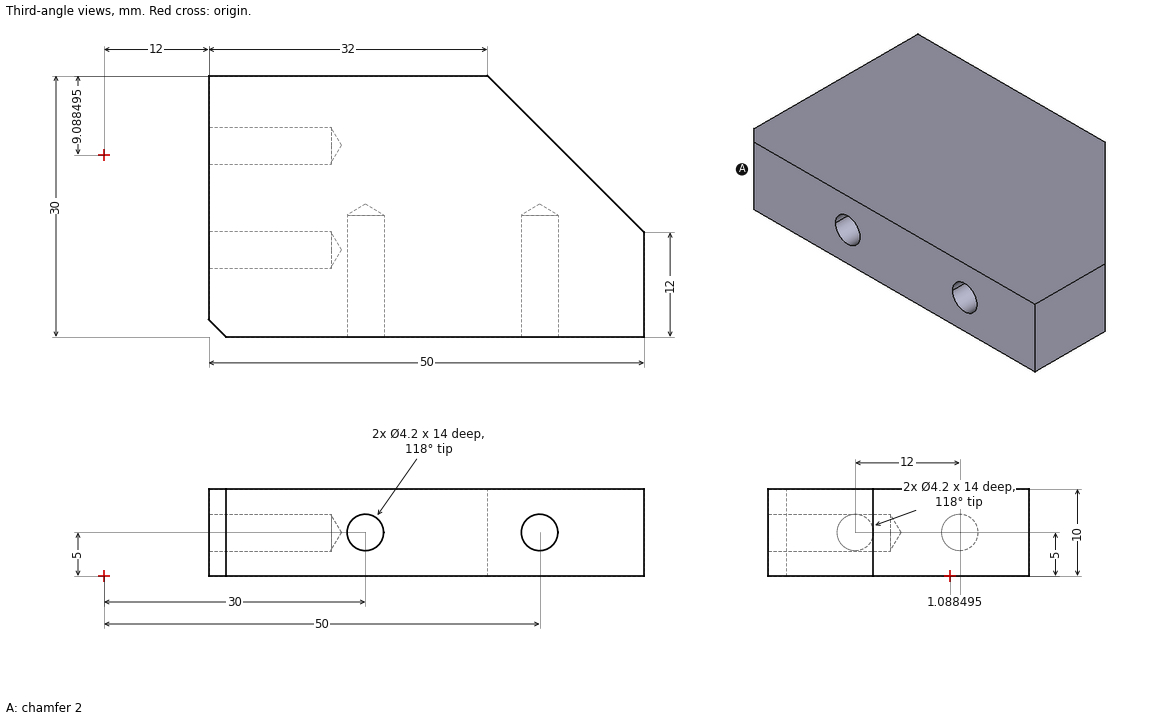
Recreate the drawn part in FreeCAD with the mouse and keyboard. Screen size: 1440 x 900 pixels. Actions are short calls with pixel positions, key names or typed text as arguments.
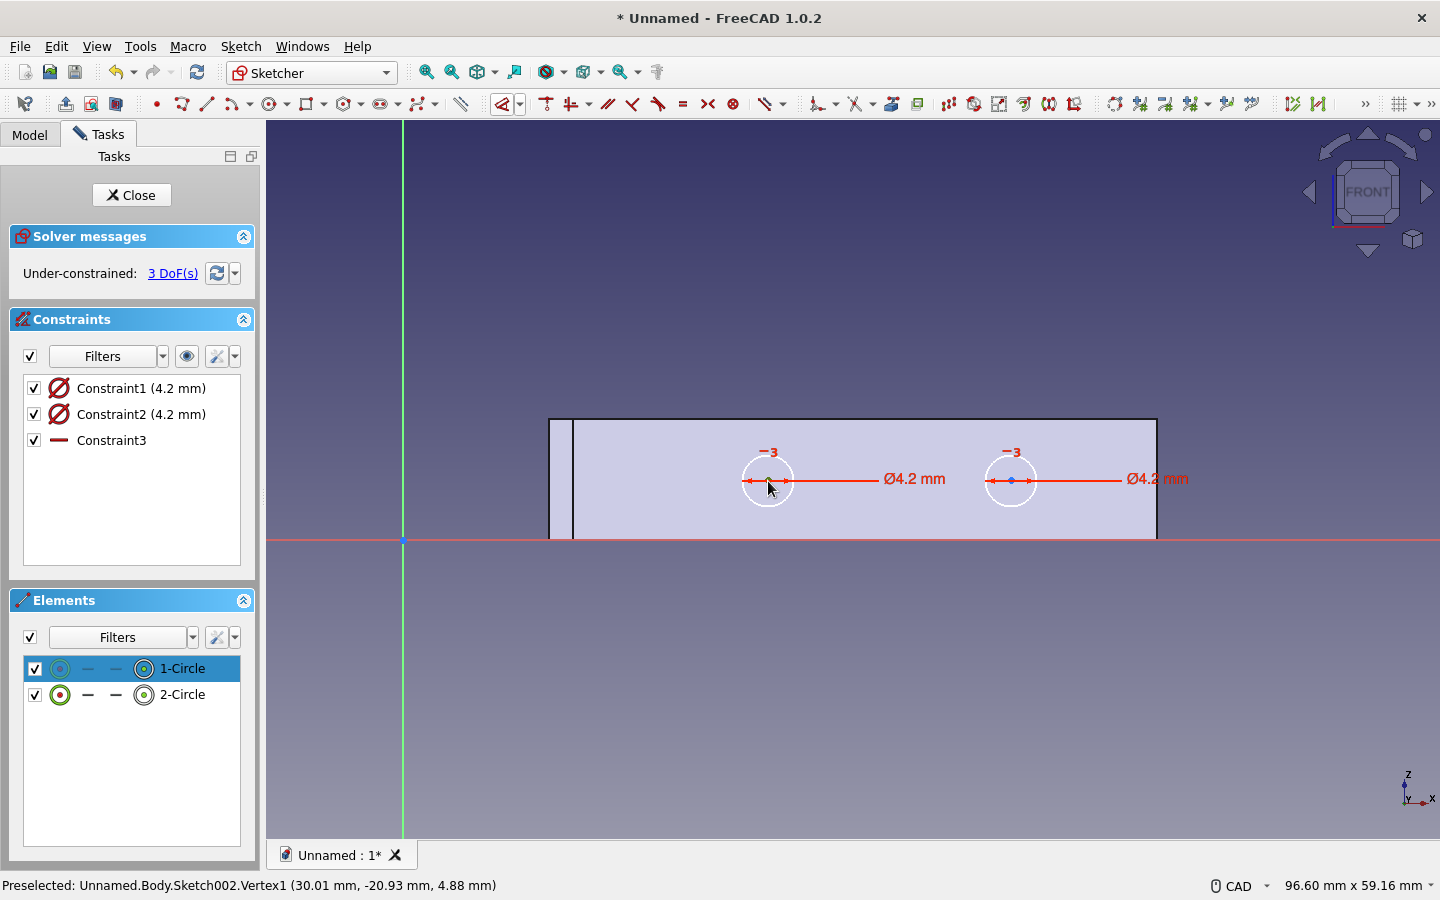
key(i)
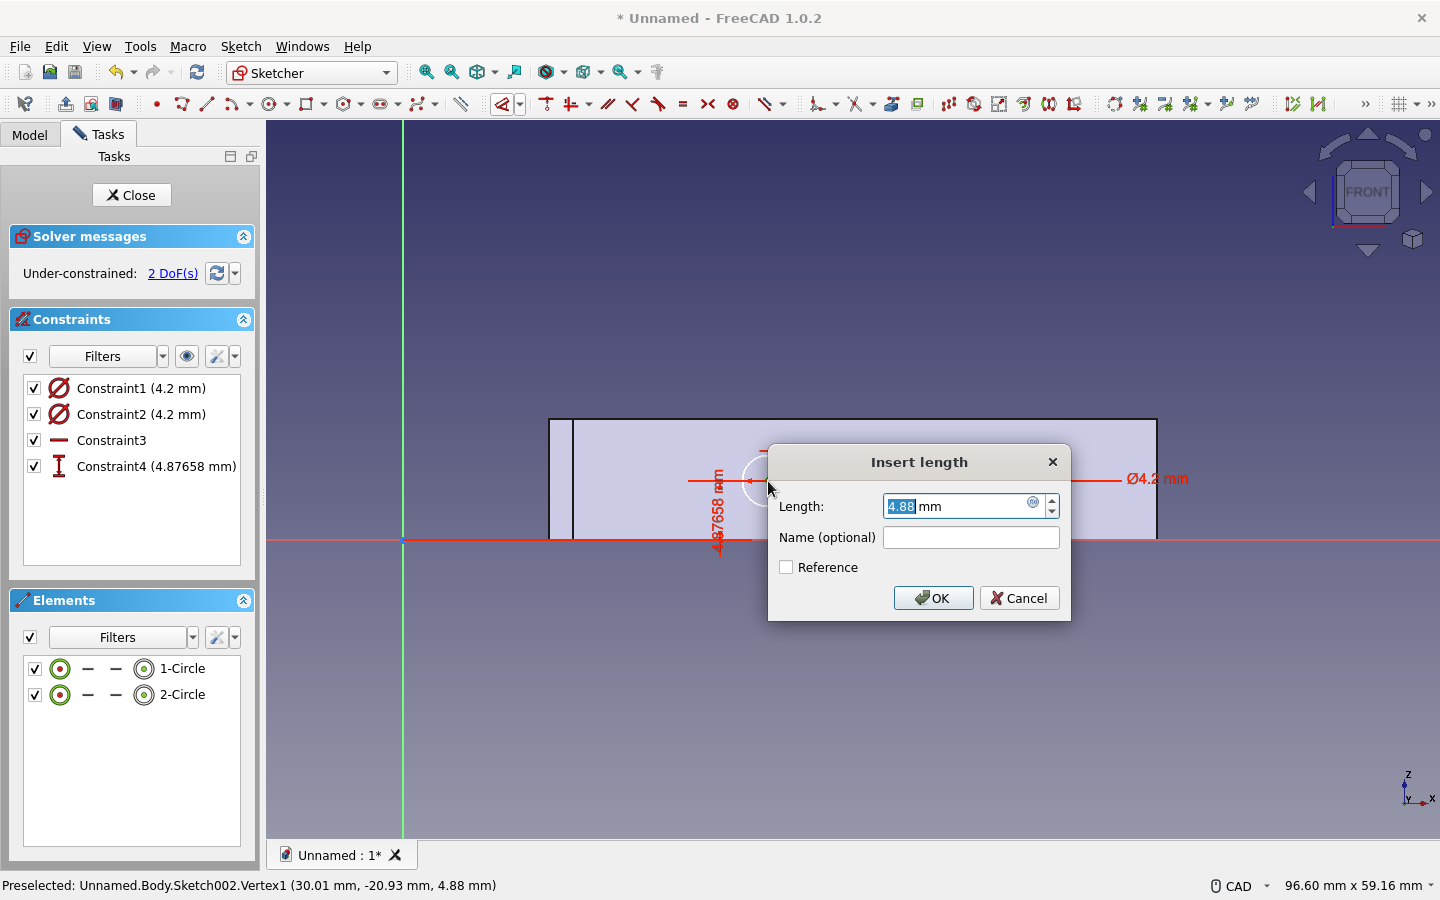
text(5)
key(Return)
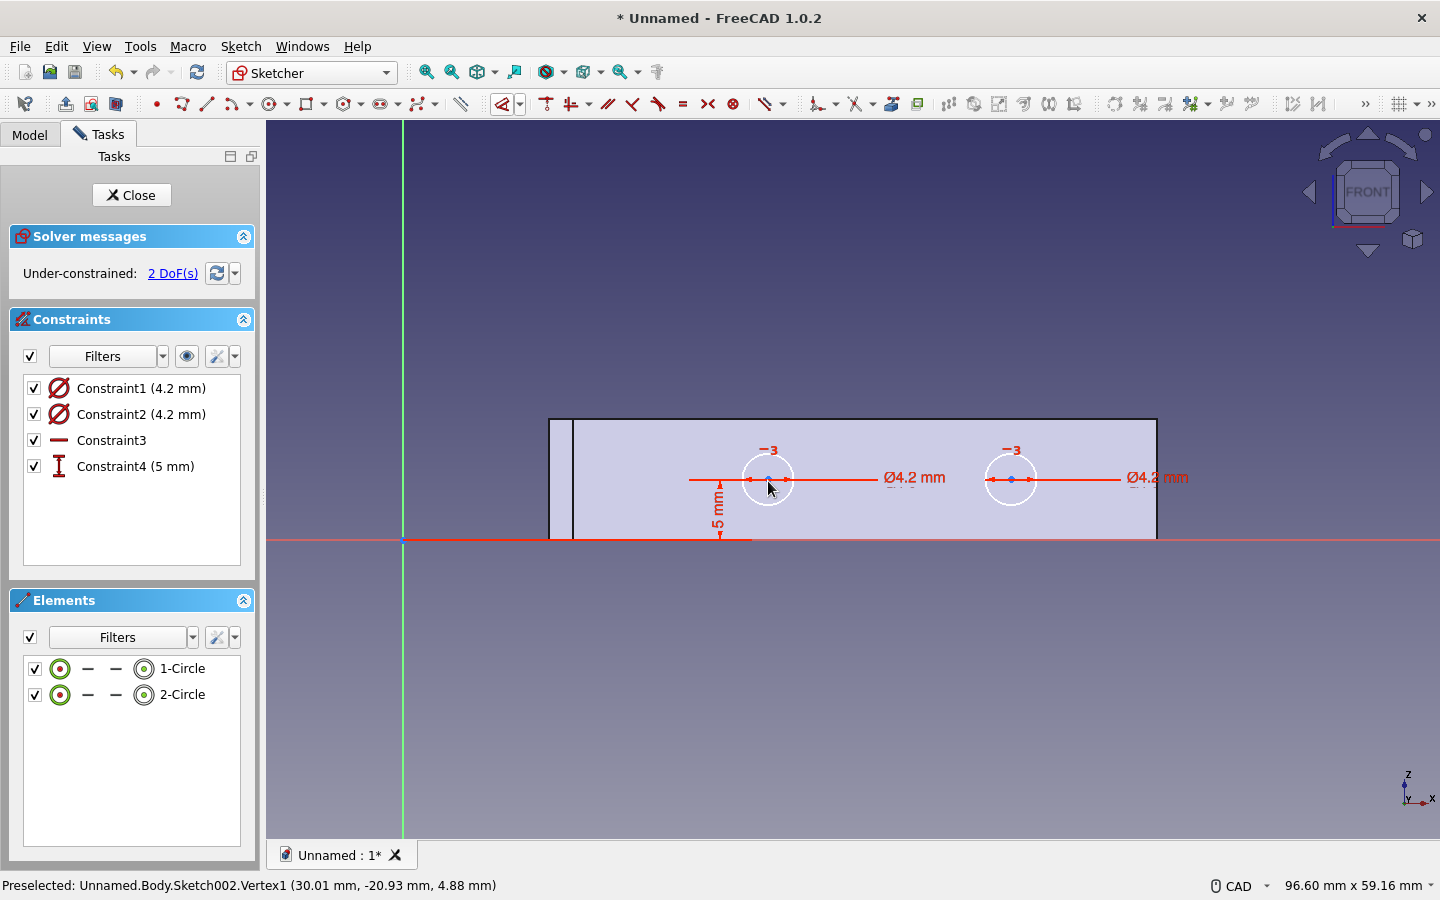
click(768, 480)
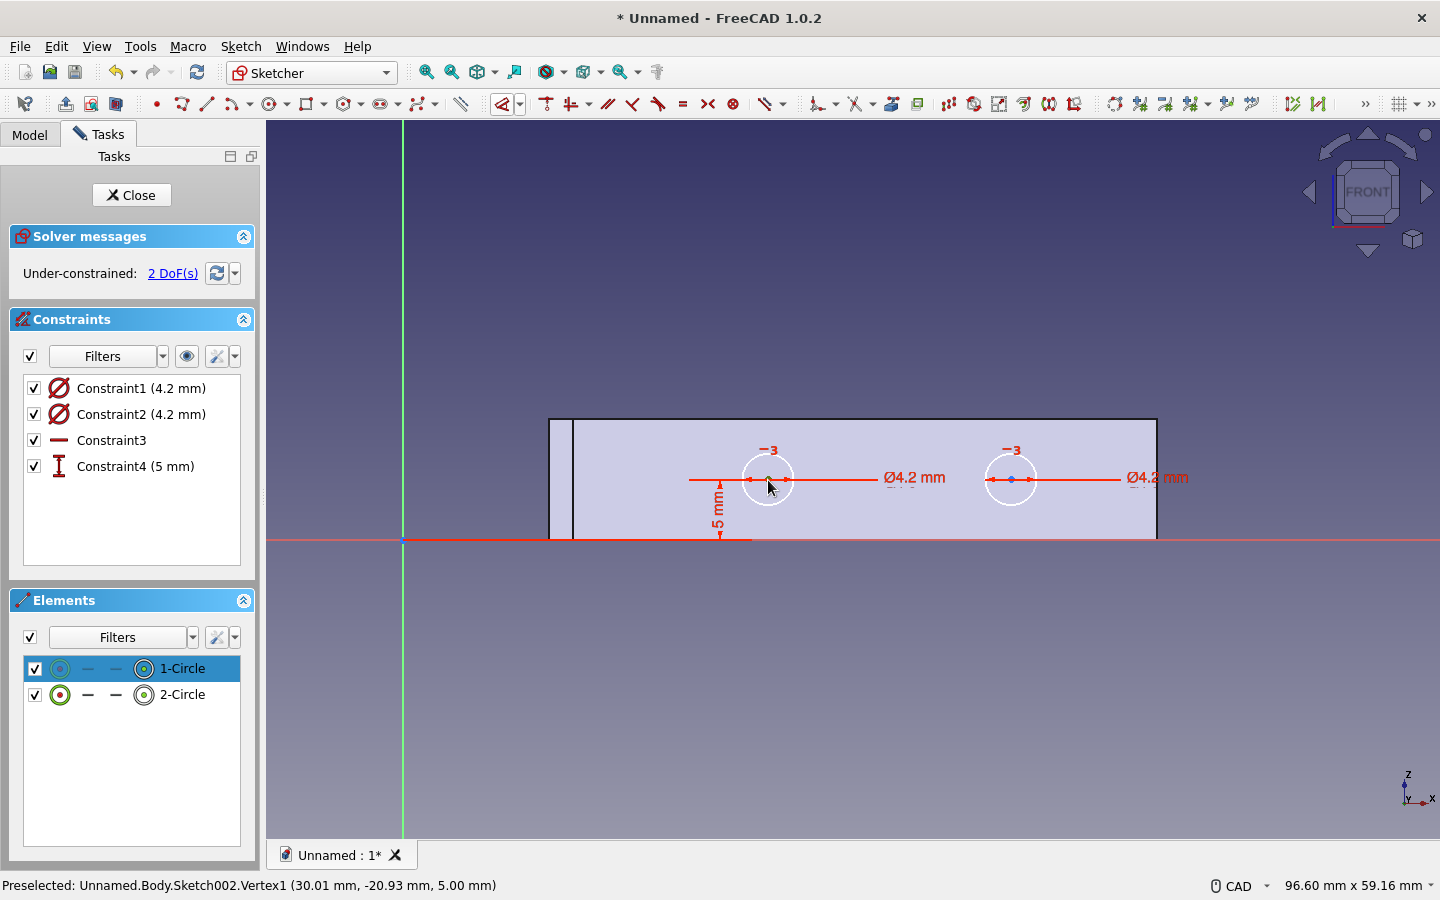
click(520, 104)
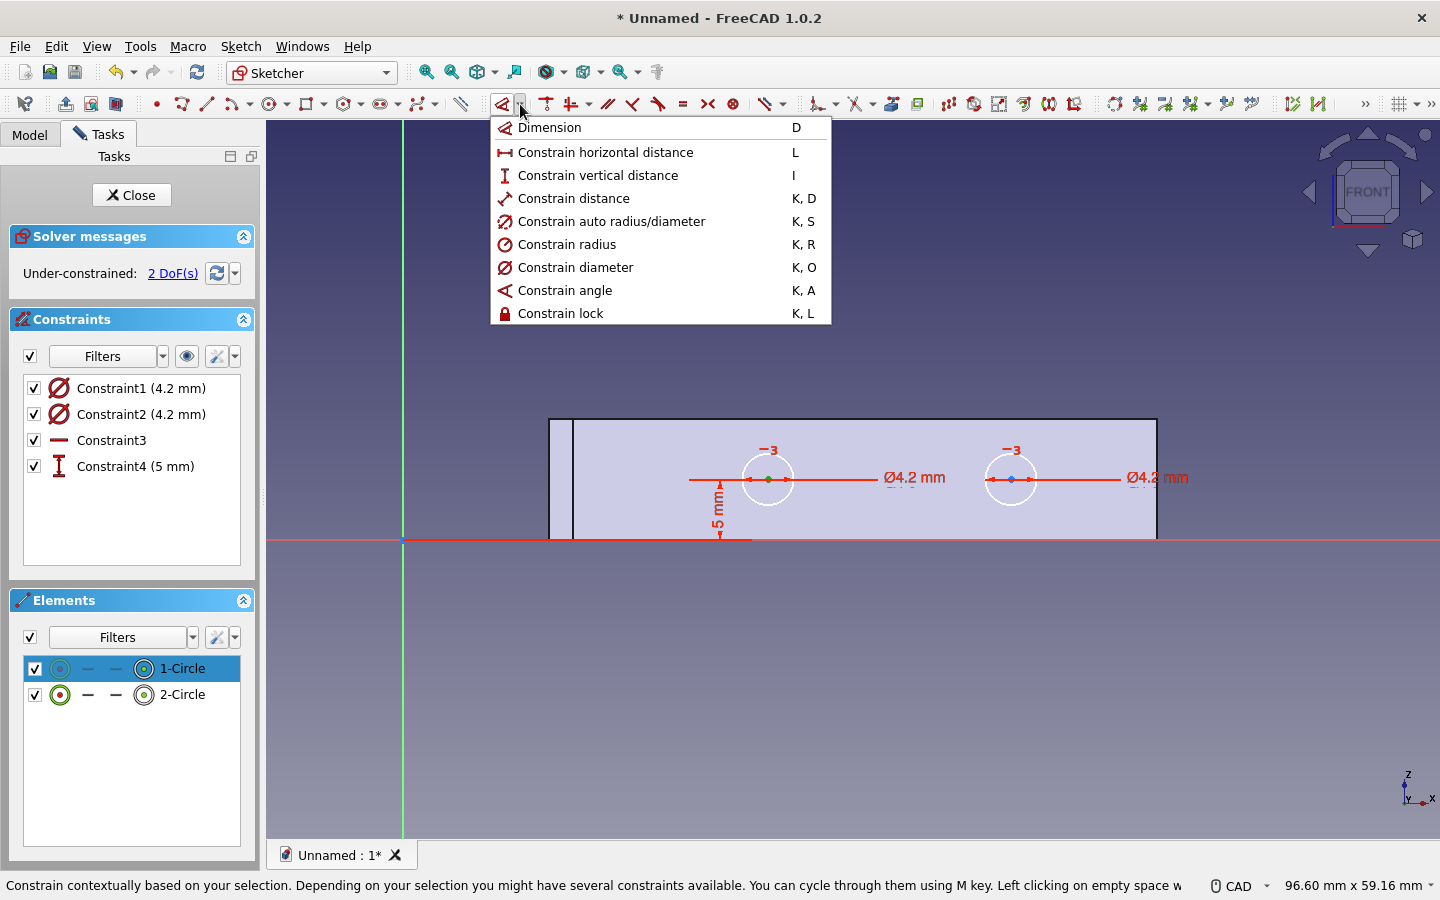
click(661, 152)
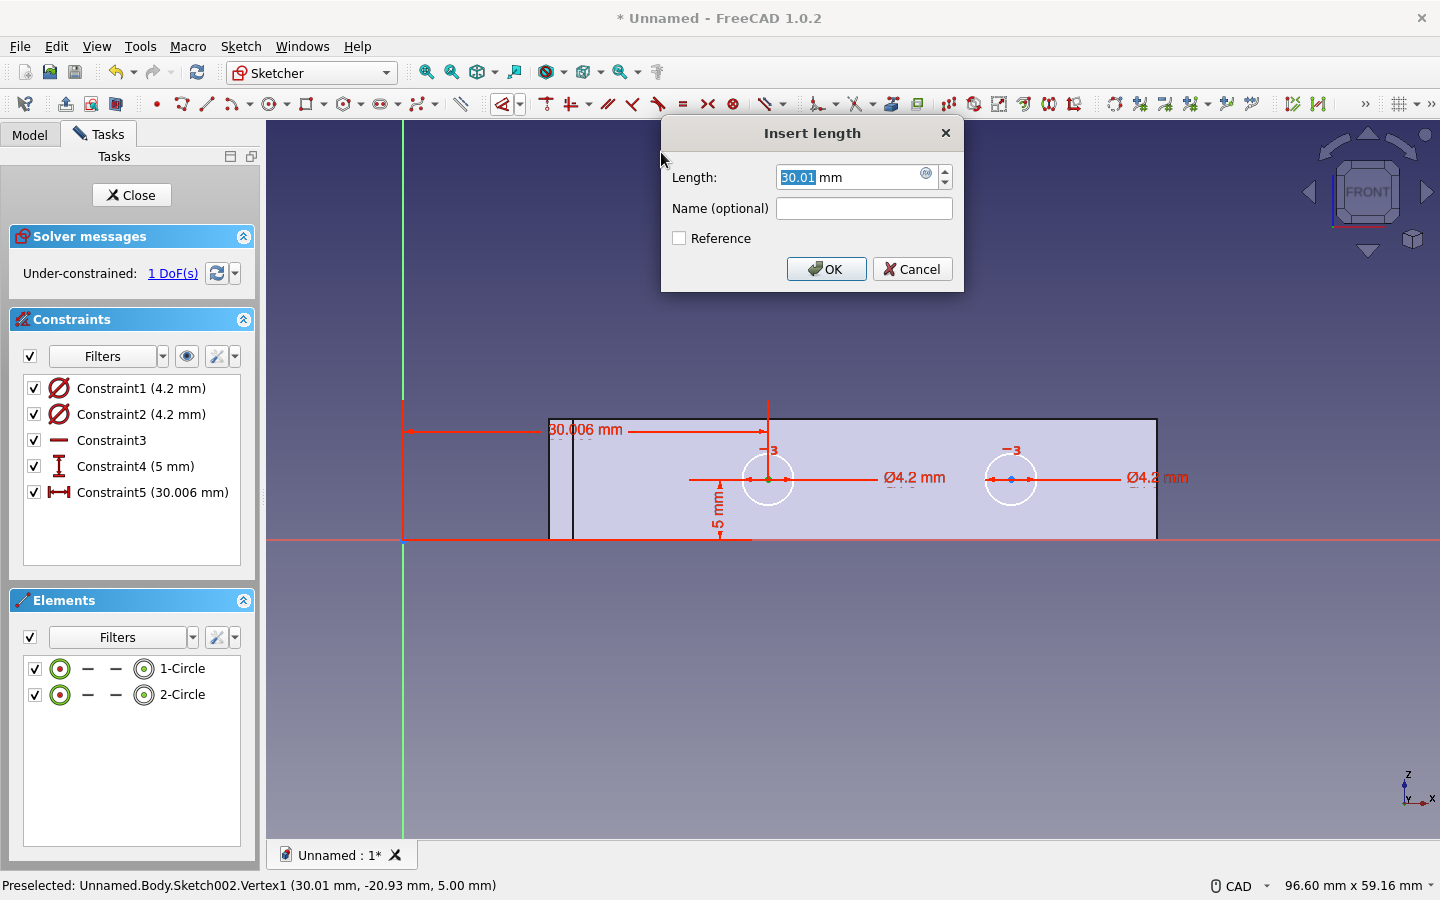
text(30)
key(Return)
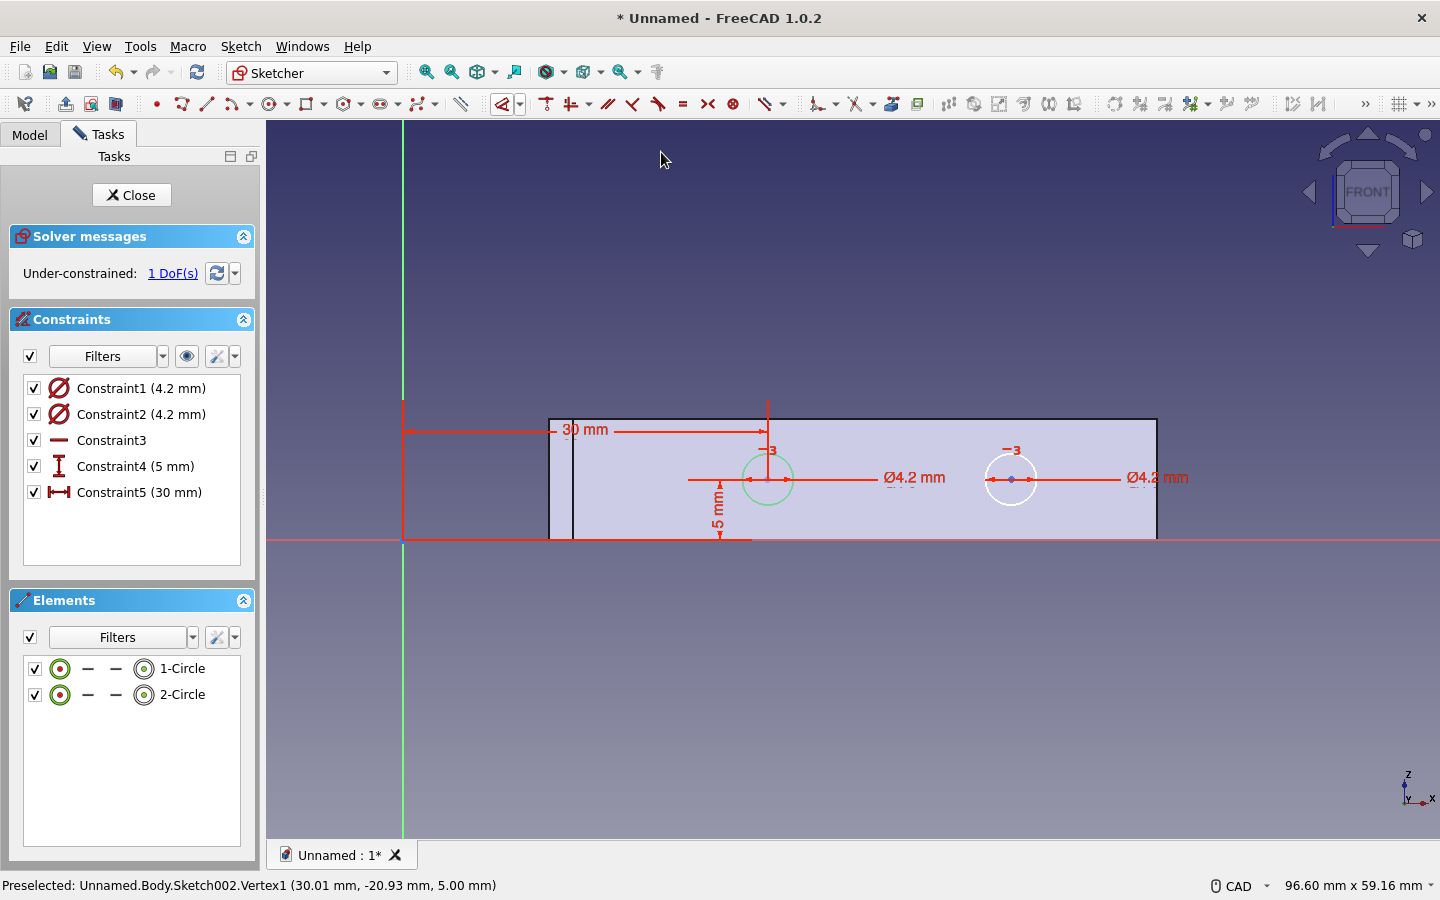
click(1011, 480)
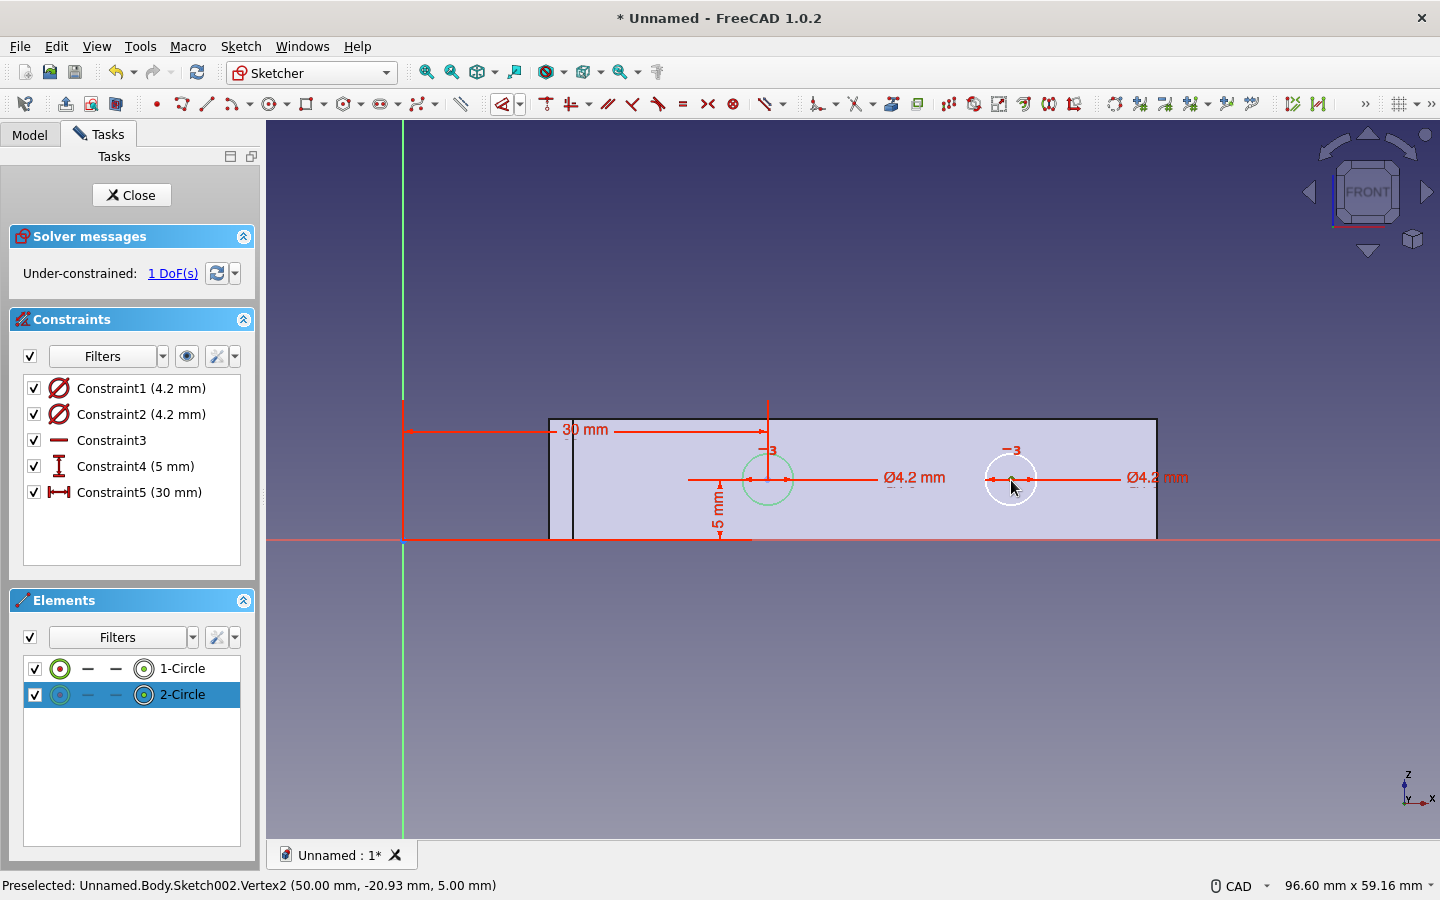
click(520, 104)